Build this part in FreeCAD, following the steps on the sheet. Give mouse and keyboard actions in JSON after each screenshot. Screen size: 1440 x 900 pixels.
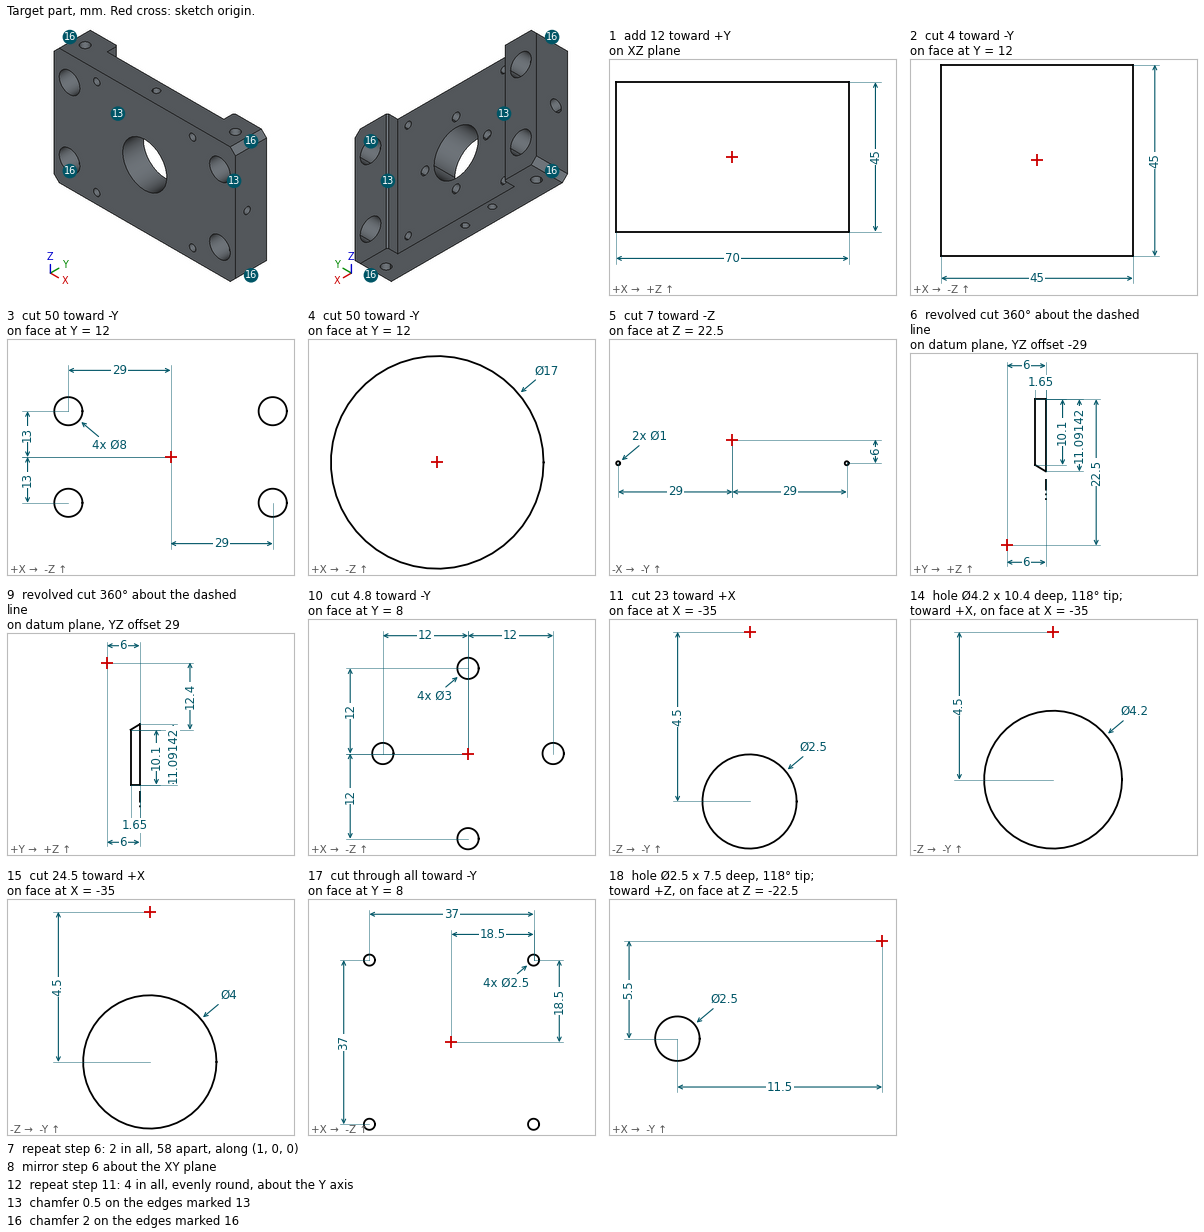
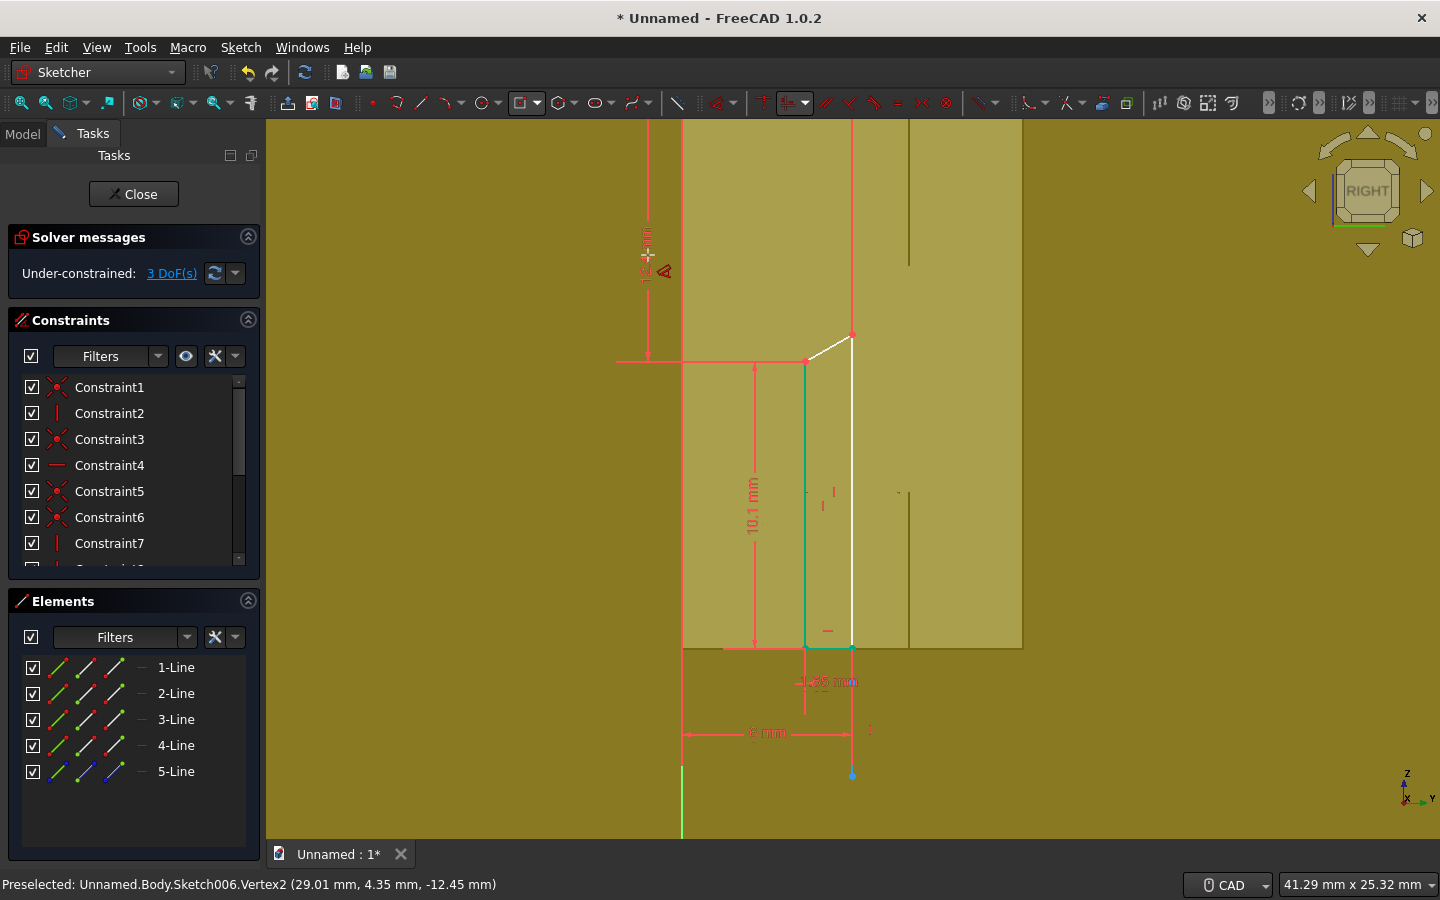
{"action": "left_click", "coordinate": [852, 555]}
{"action": "left_click", "coordinate": [886, 492]}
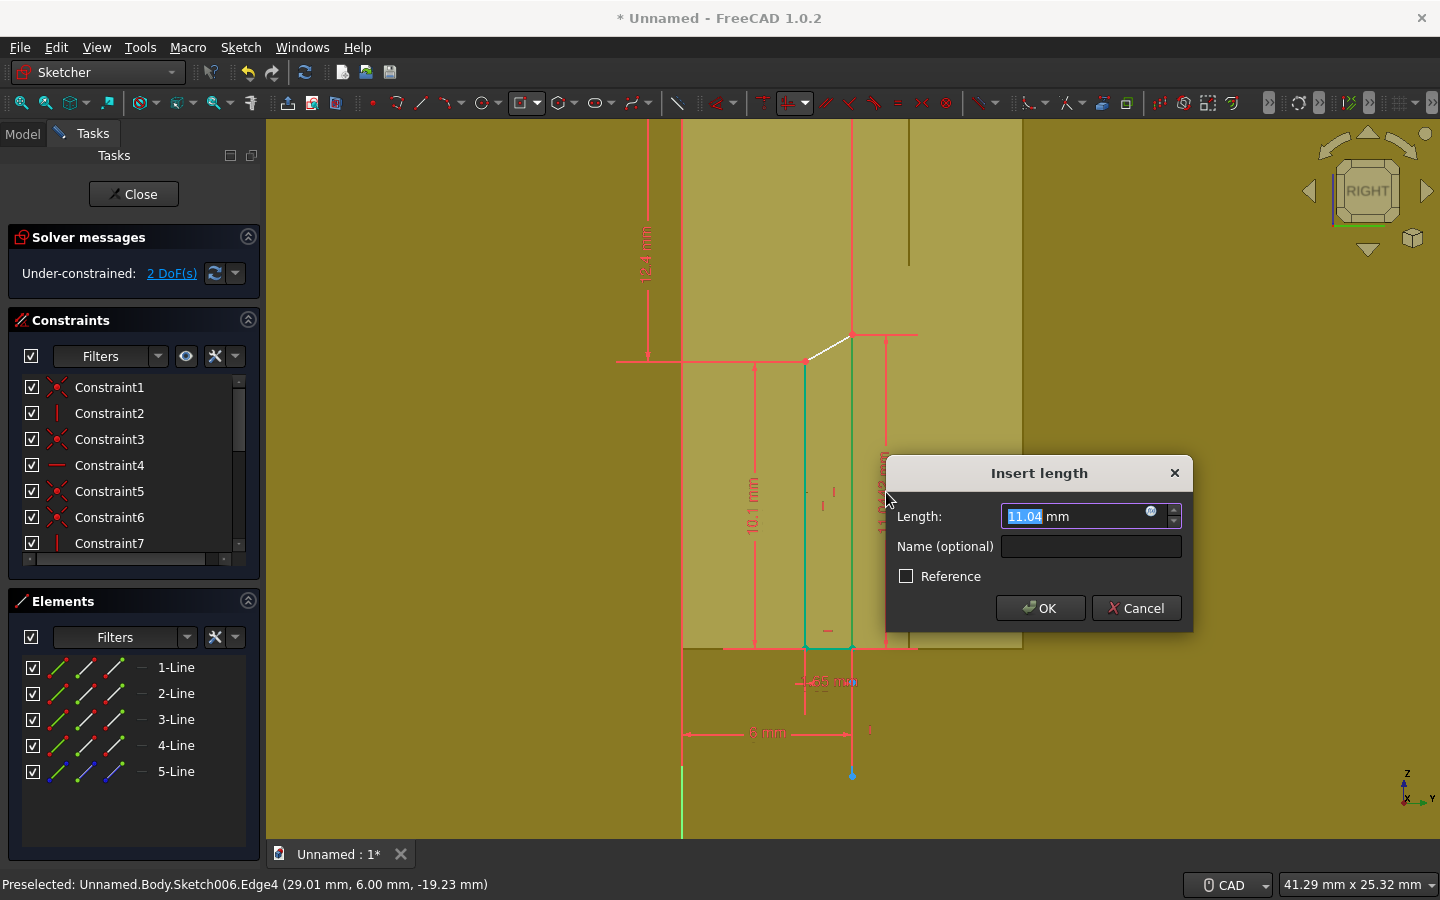
{"action": "type", "text": "11.09142"}
{"action": "key", "text": "Return"}
{"action": "key", "text": "Escape"}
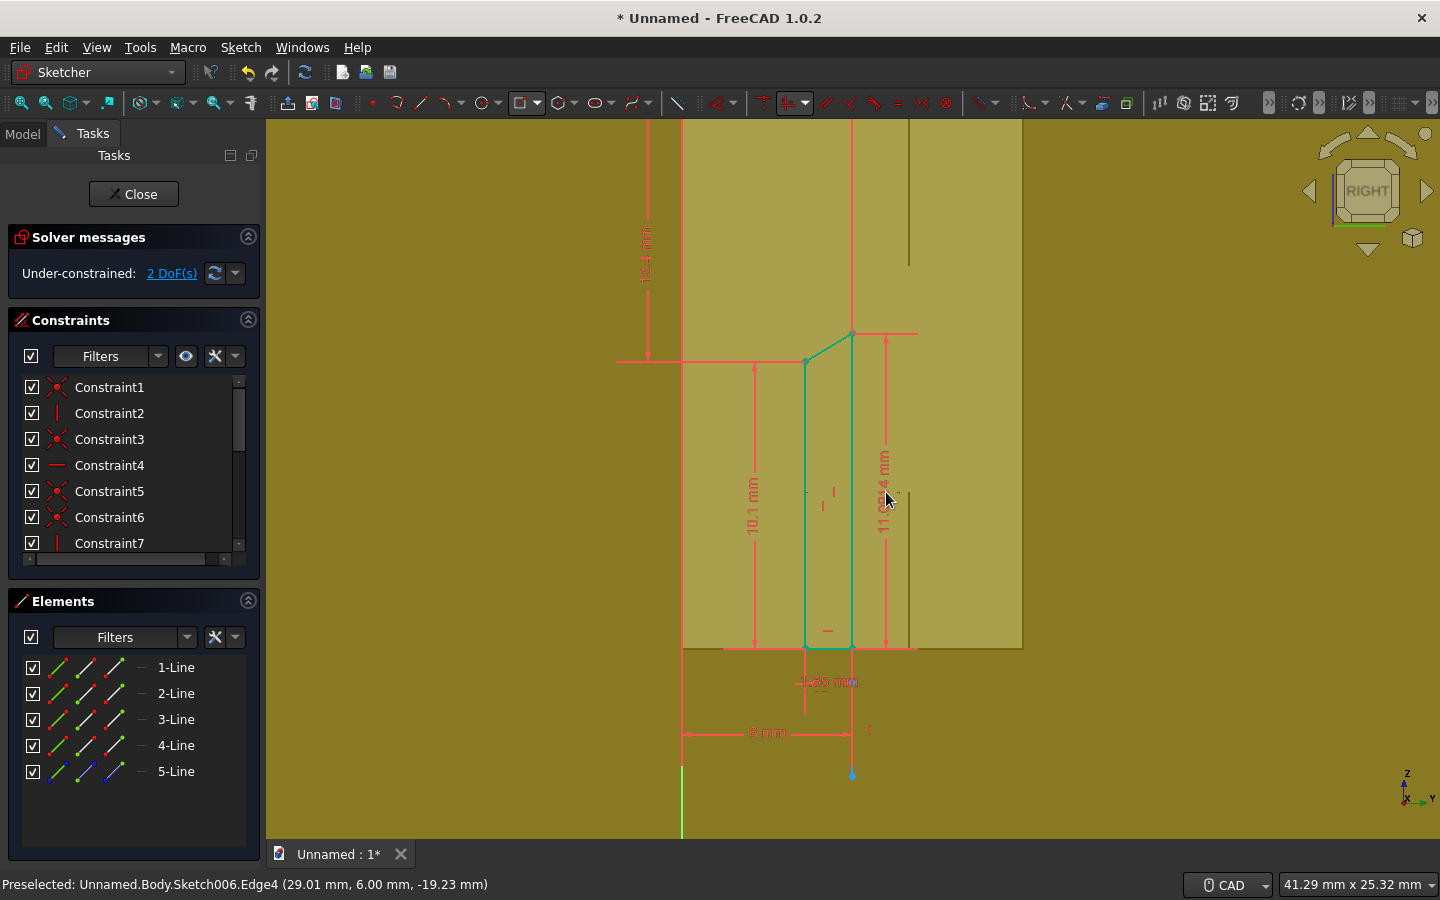
{"action": "left_click", "coordinate": [134, 194]}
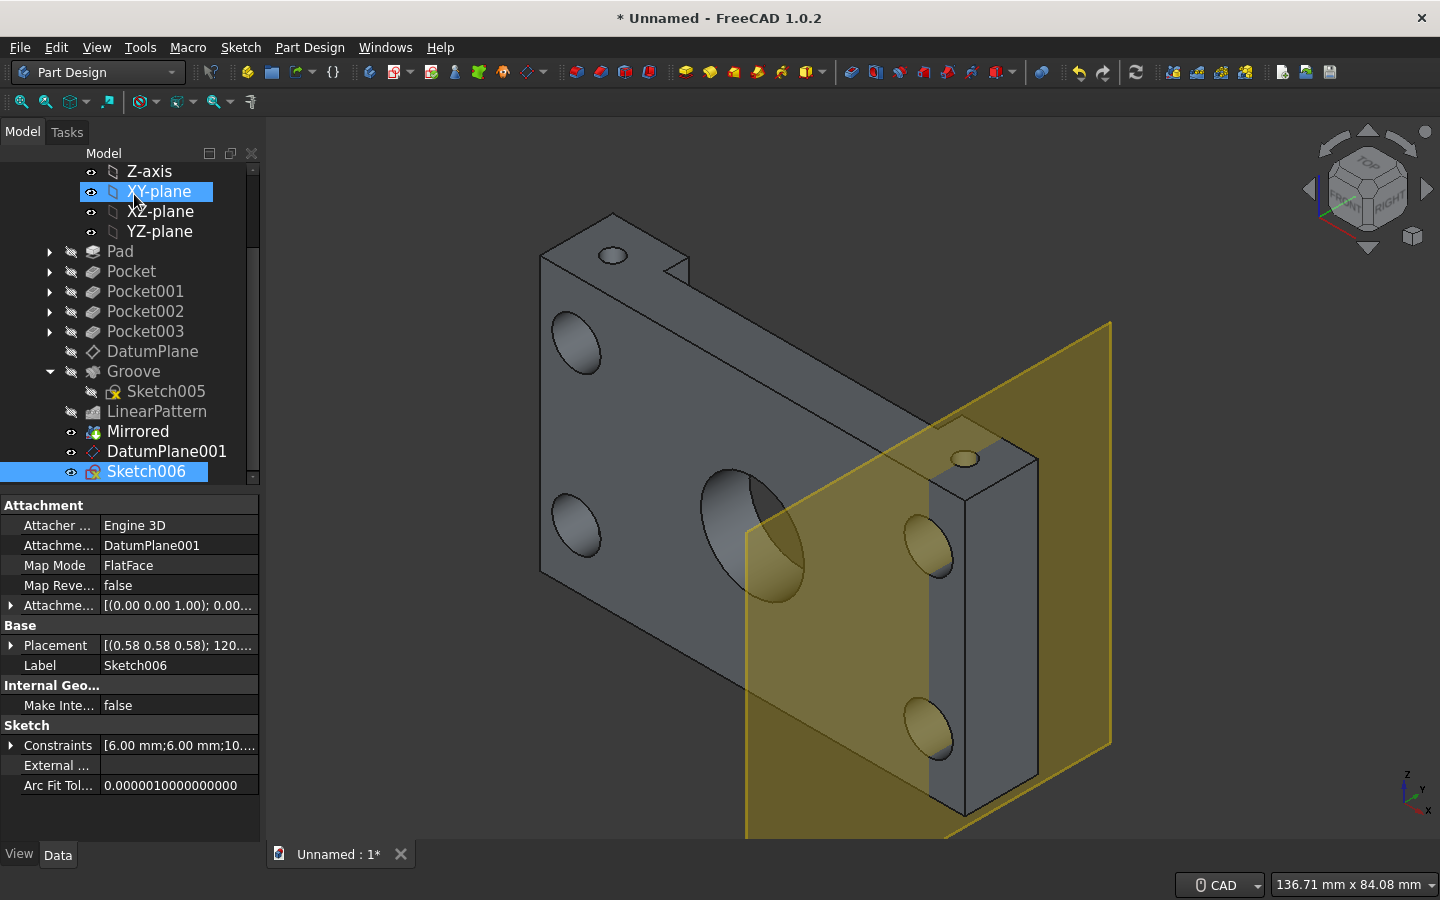
{"action": "left_click", "coordinate": [900, 72]}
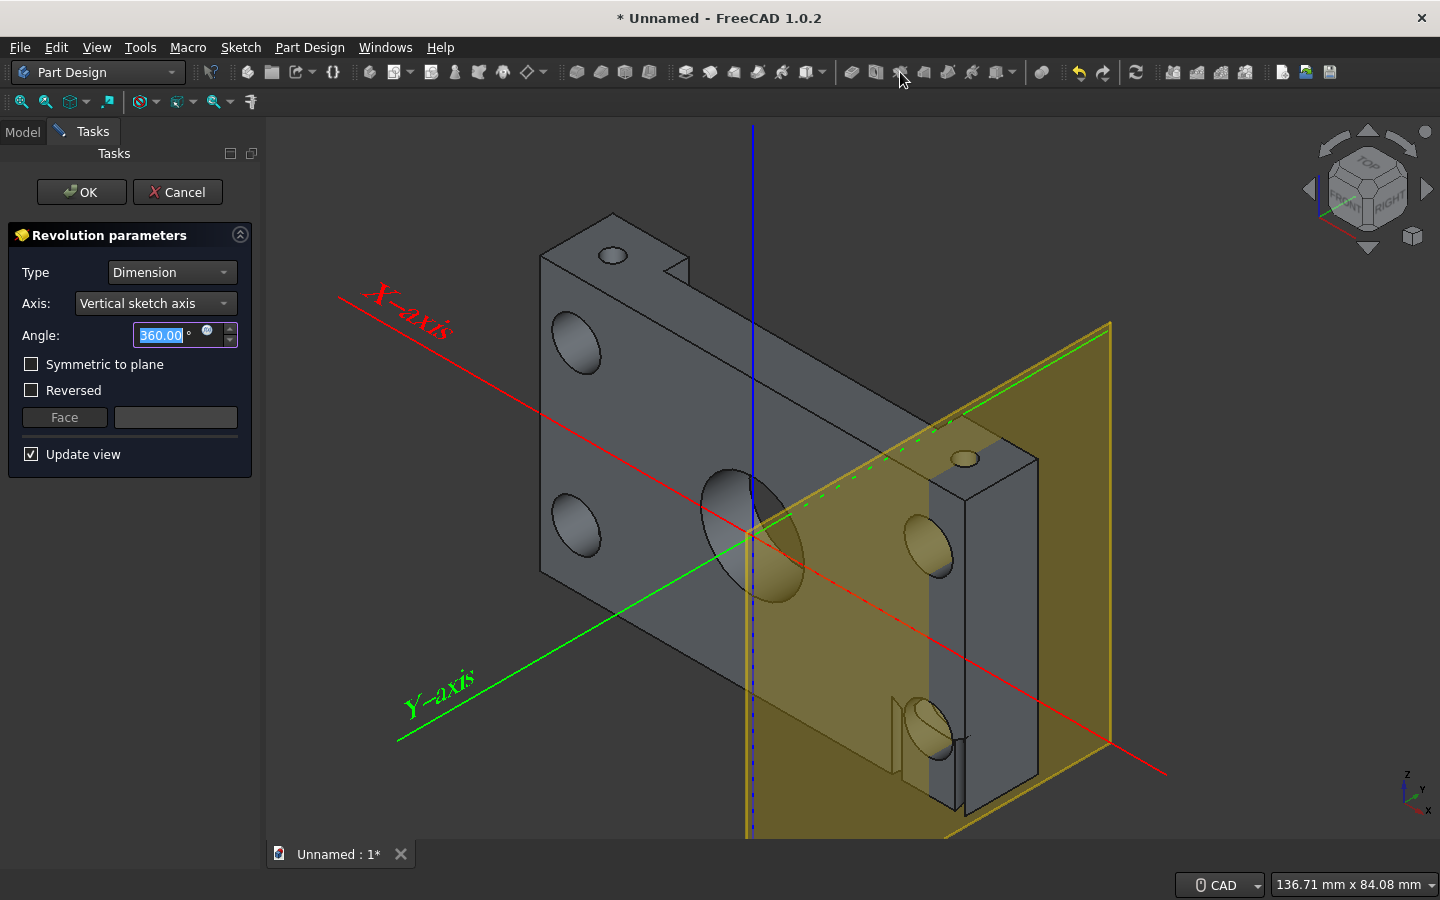
{"action": "left_click", "coordinate": [156, 304]}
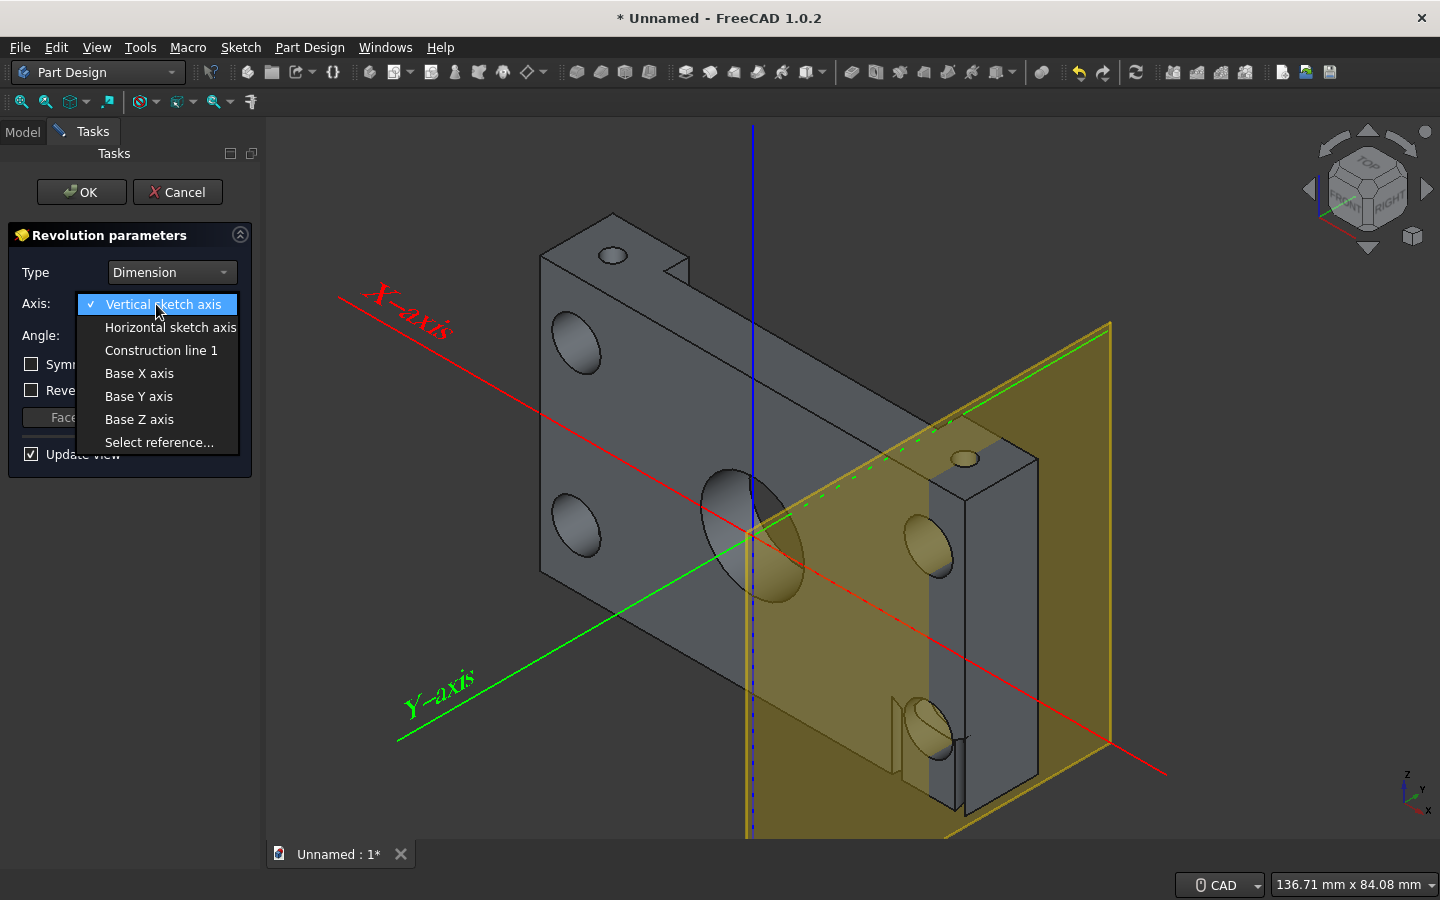
{"action": "left_click", "coordinate": [156, 350]}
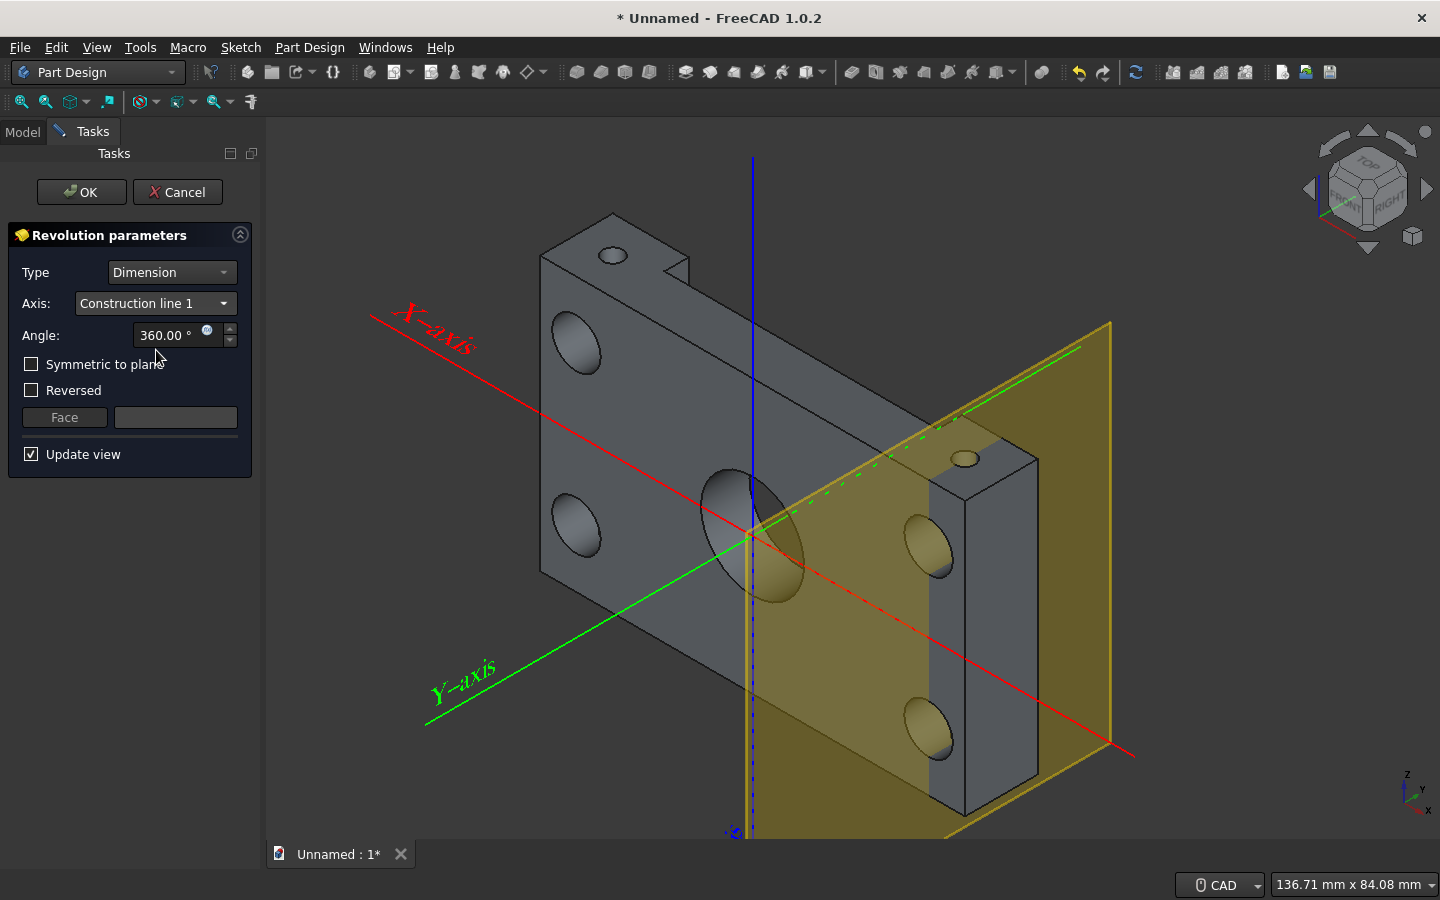
{"action": "left_click", "coordinate": [82, 192]}